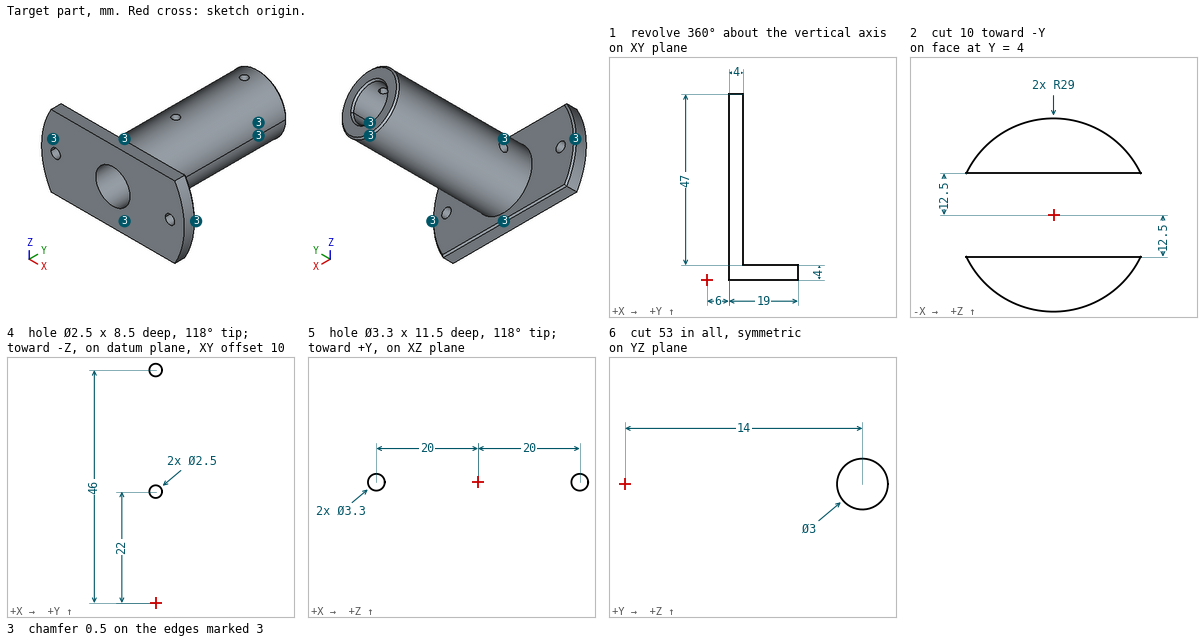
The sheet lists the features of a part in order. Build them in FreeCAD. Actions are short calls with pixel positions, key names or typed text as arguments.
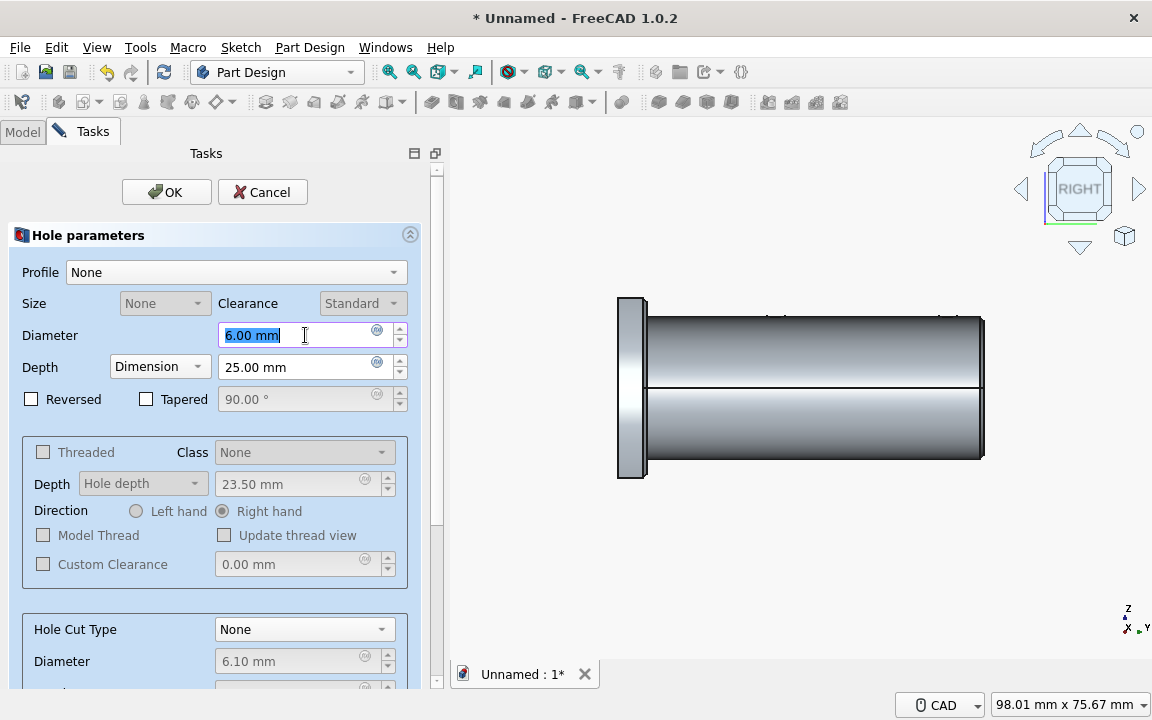
text(3.3)
key(Tab)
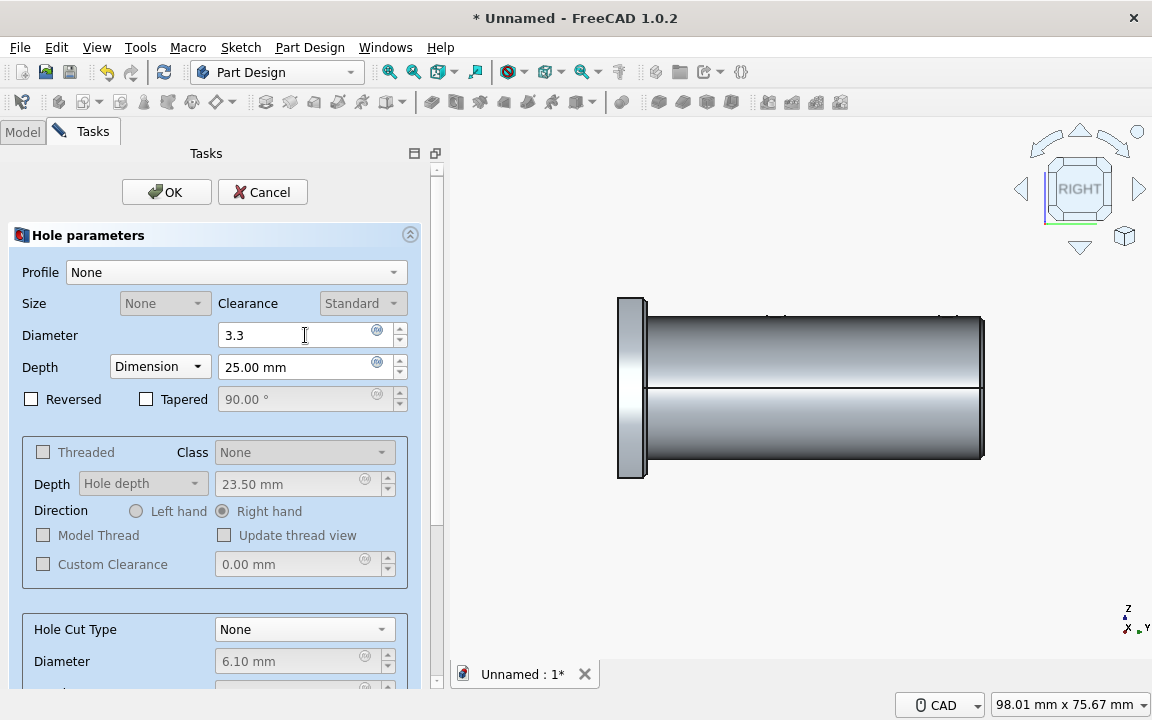
triple_click(305, 367)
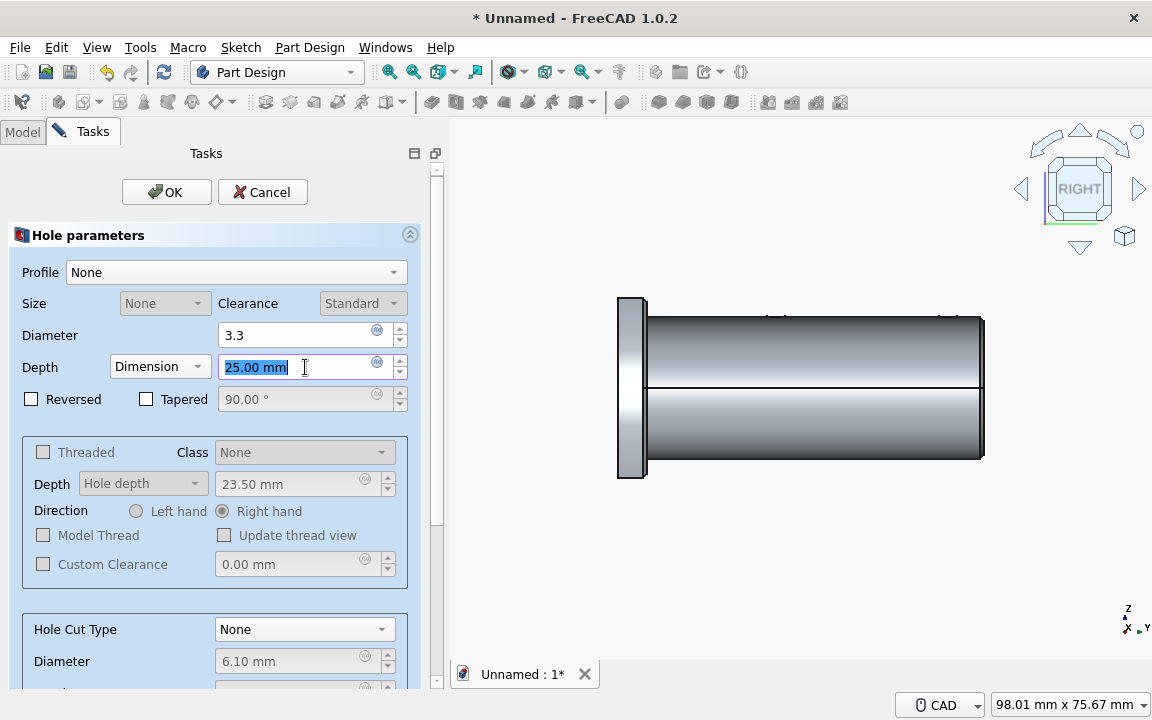
text(11.5)
key(Tab)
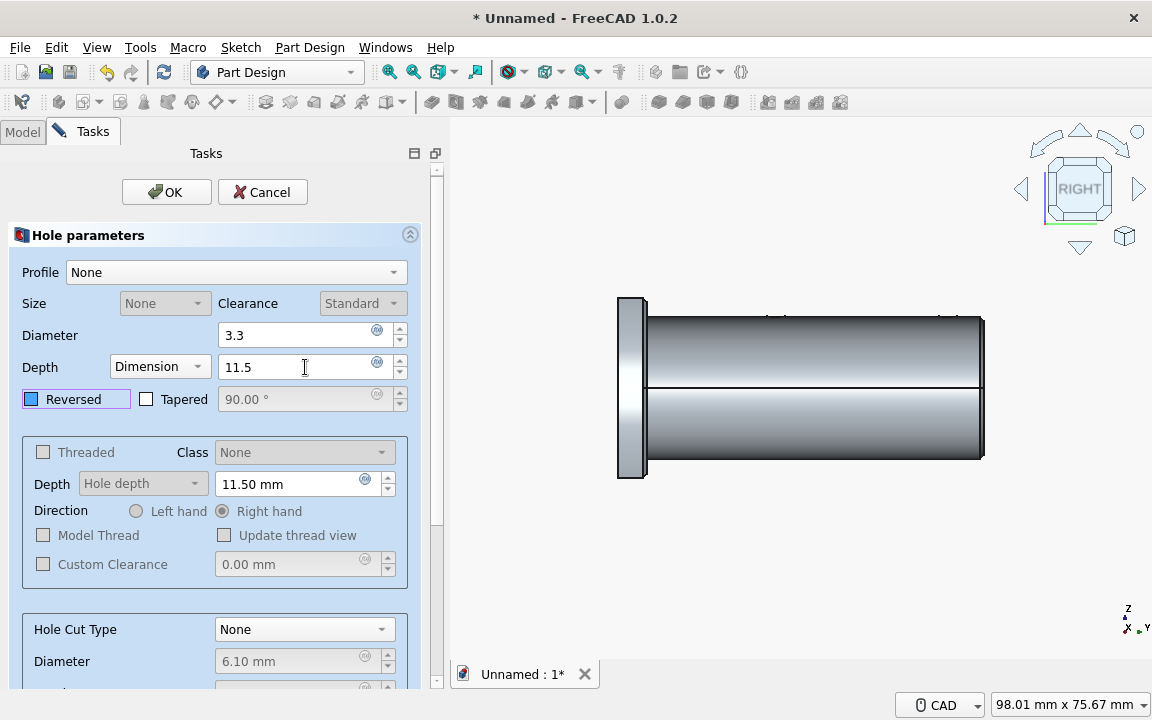
click(167, 192)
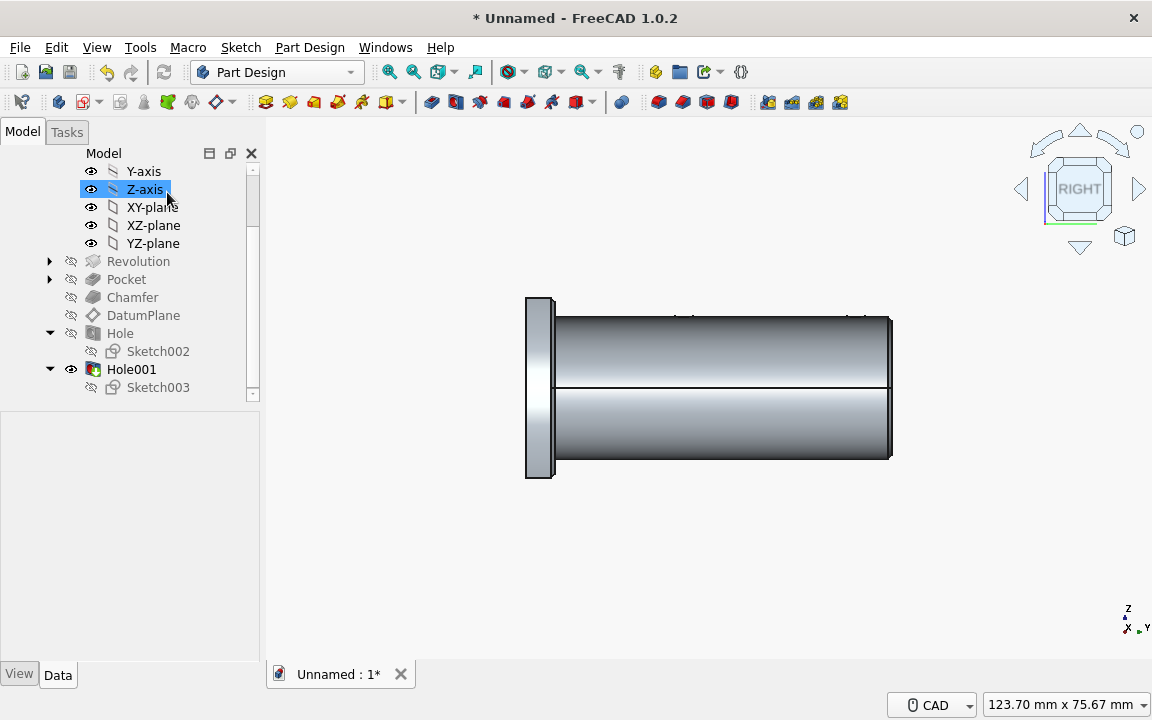
click(390, 72)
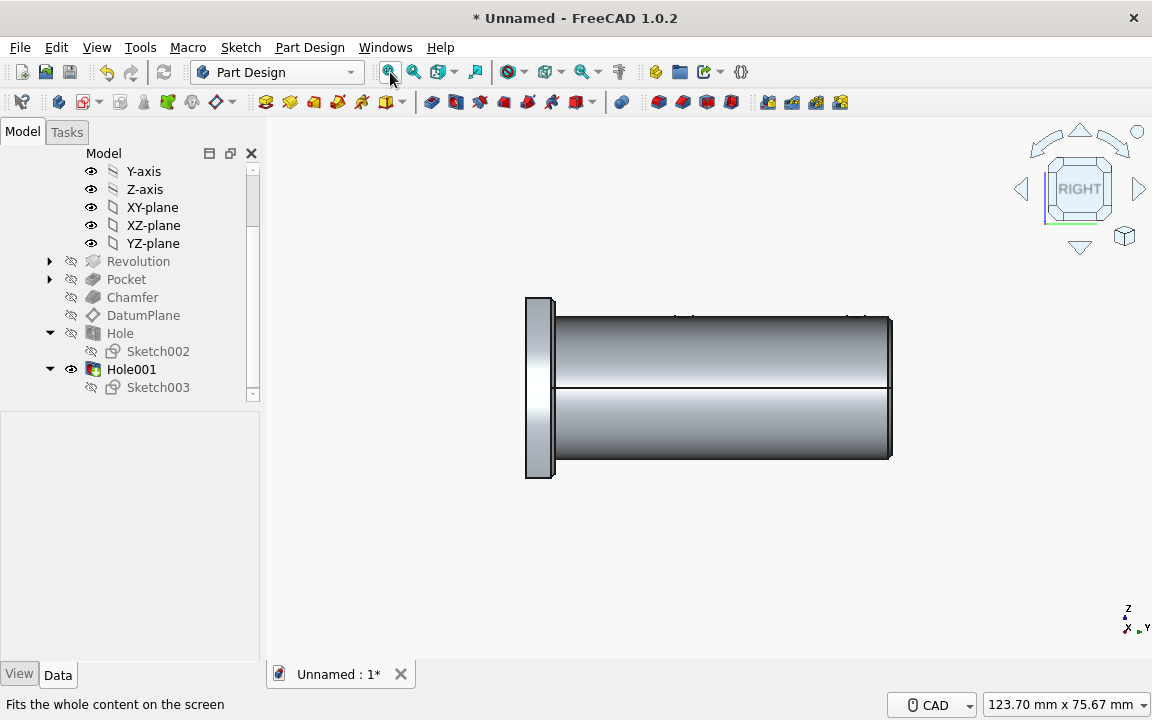
click(84, 102)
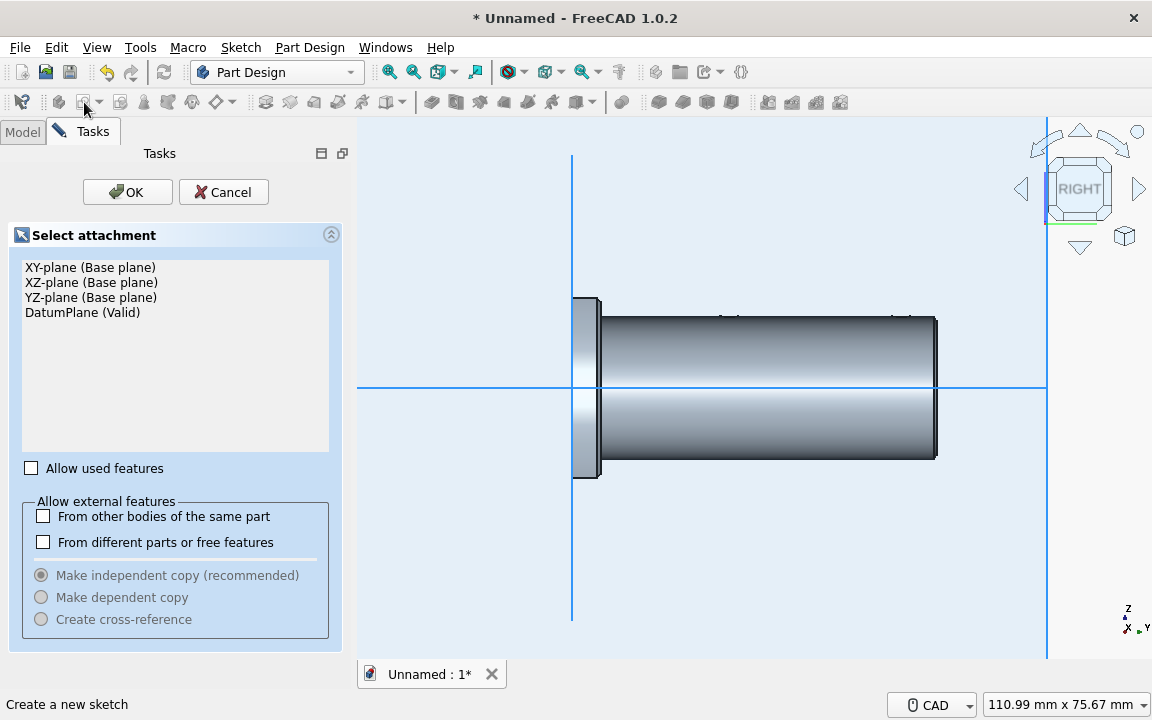
click(82, 298)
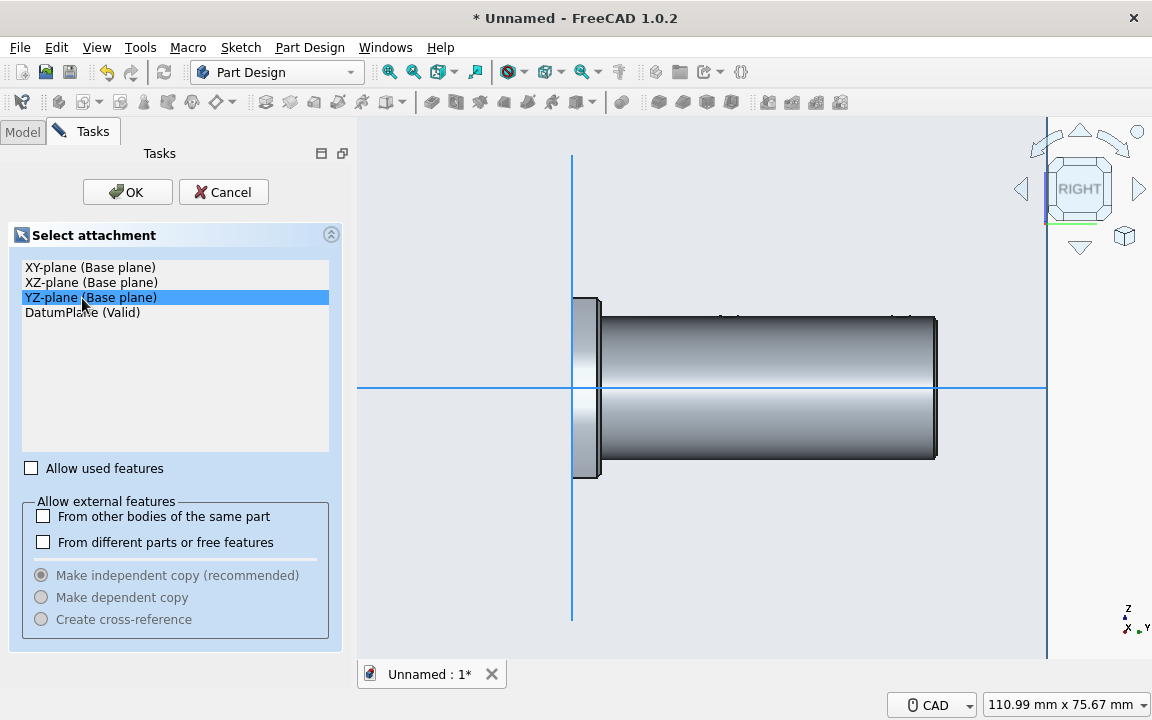
click(128, 192)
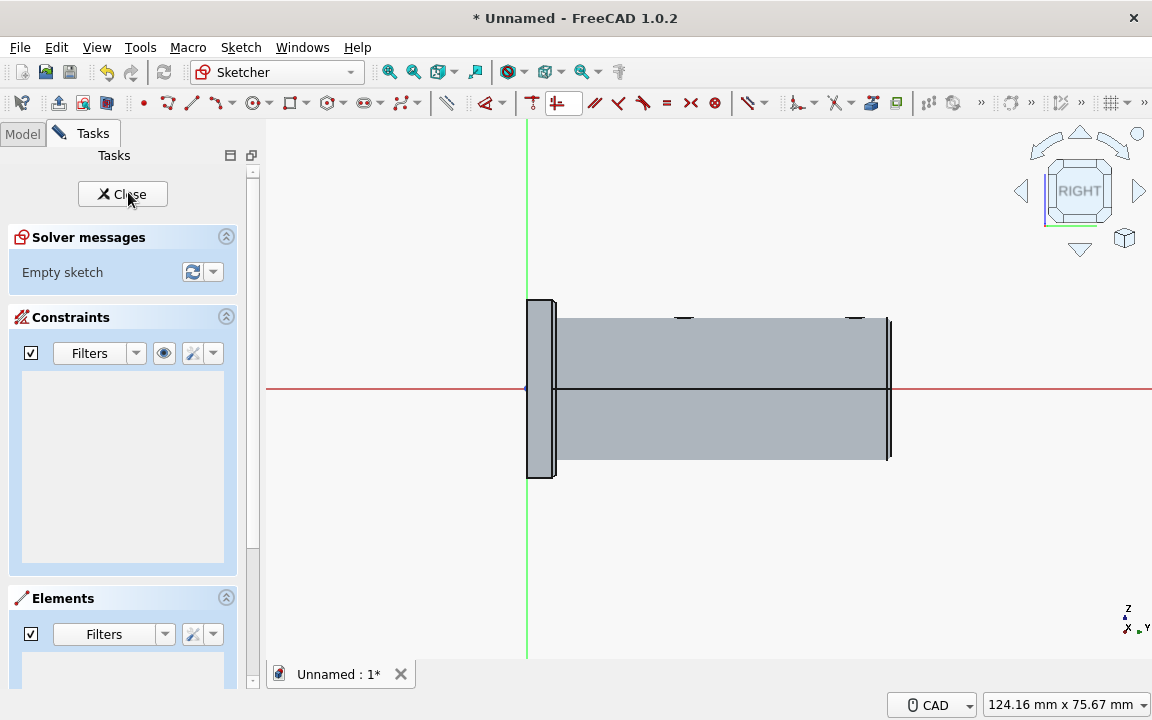
click(108, 104)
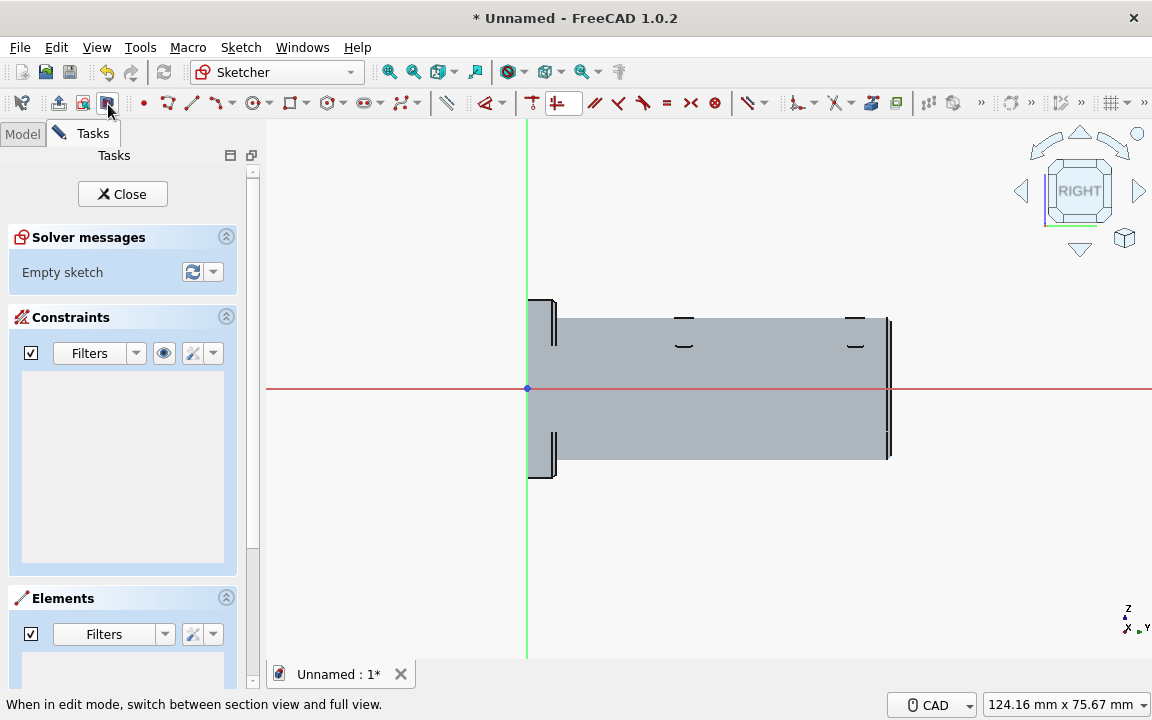
scroll(626, 389, up, 14)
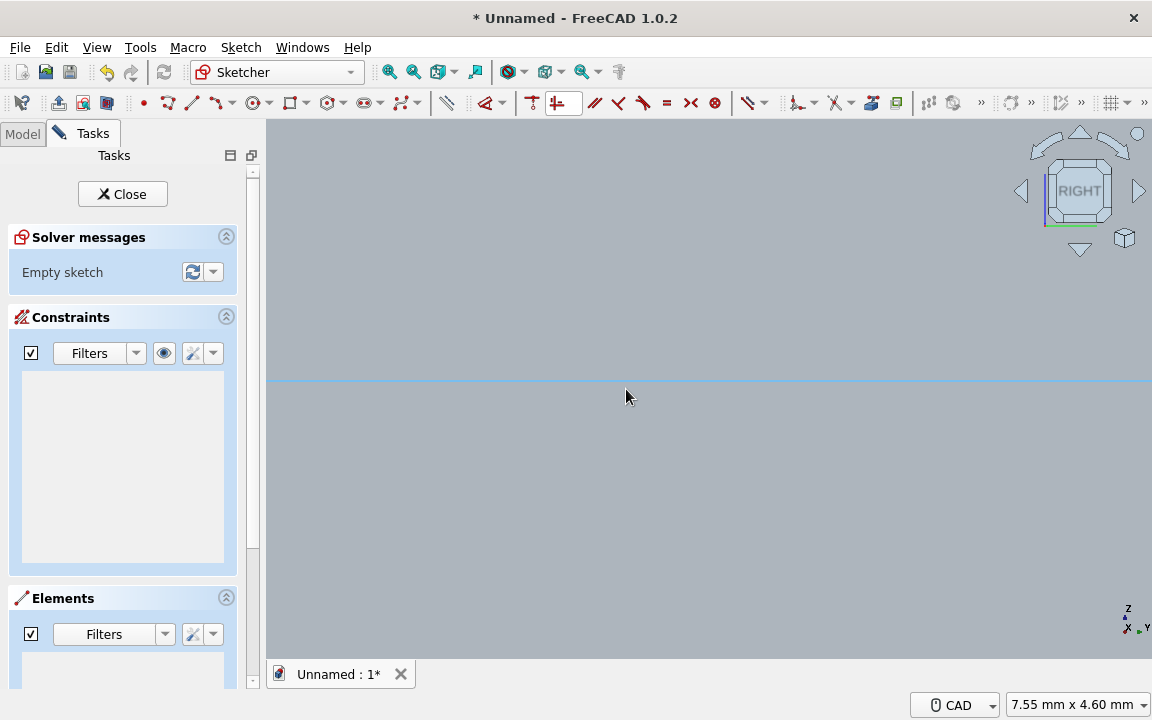
click(254, 104)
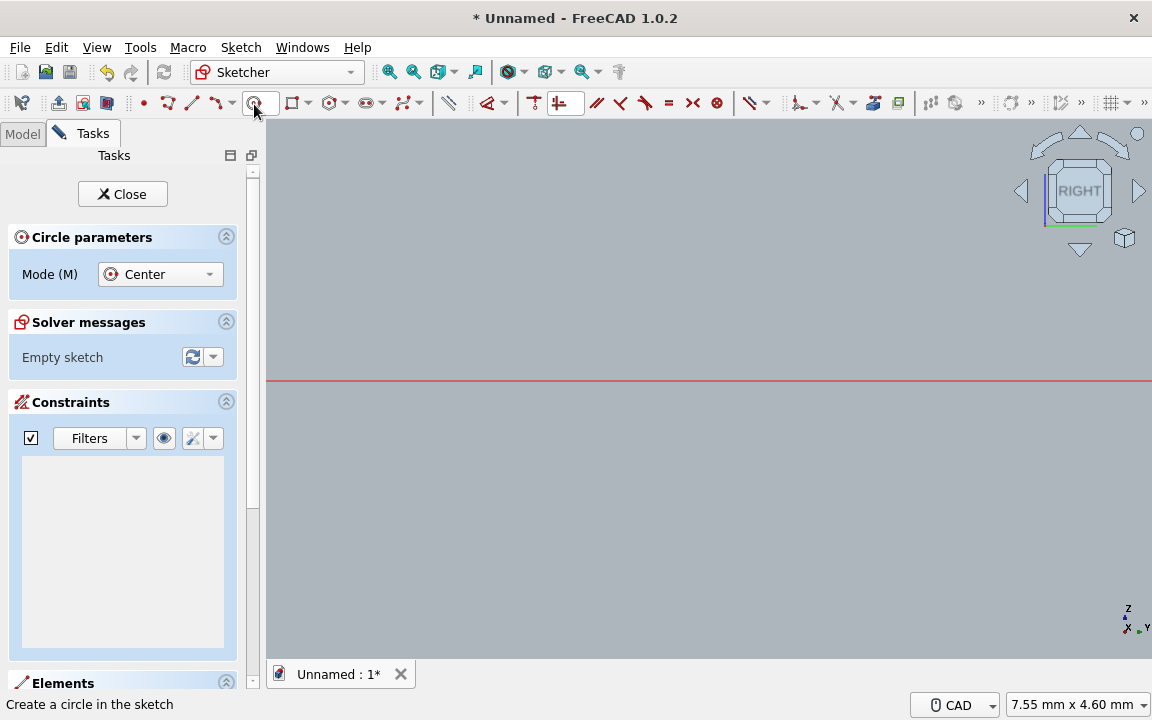
click(635, 381)
move(760, 257)